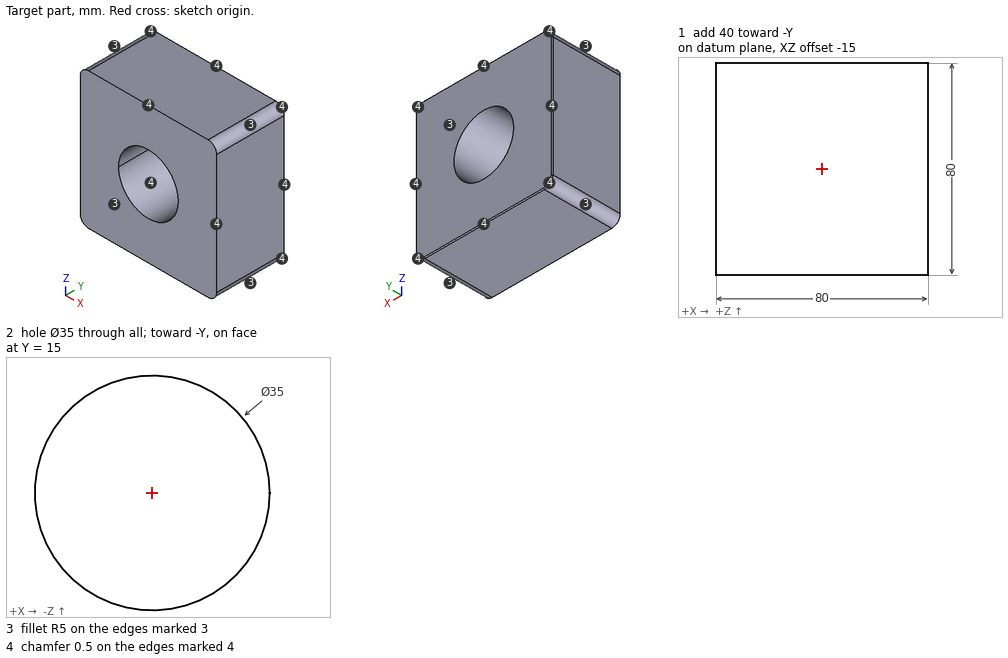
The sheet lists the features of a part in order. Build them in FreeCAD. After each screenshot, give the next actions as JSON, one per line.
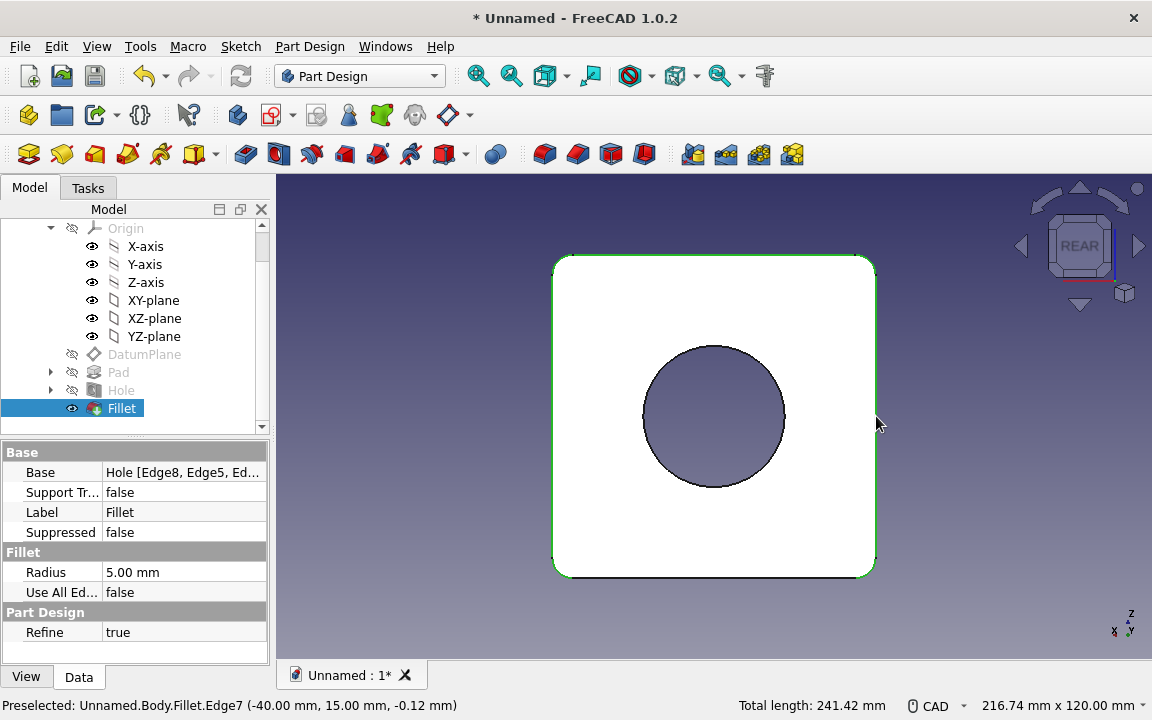
{"action": "left_click", "coordinate": [714, 577], "text": "ctrl"}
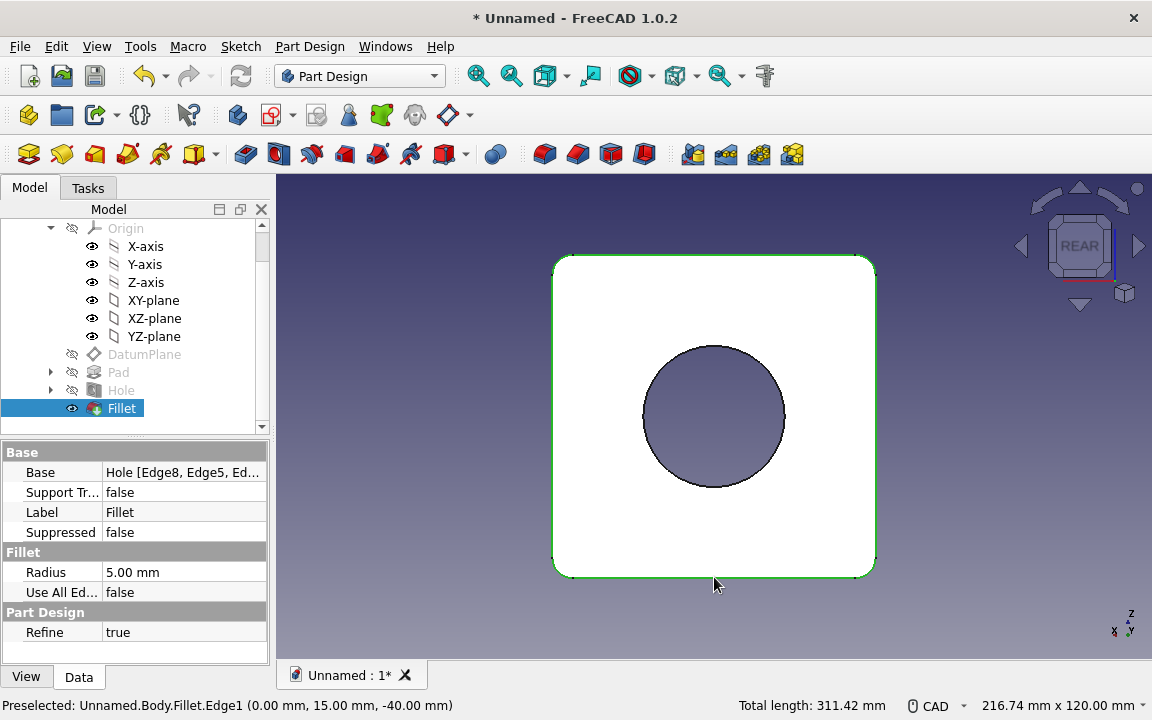
{"action": "left_click", "coordinate": [578, 154]}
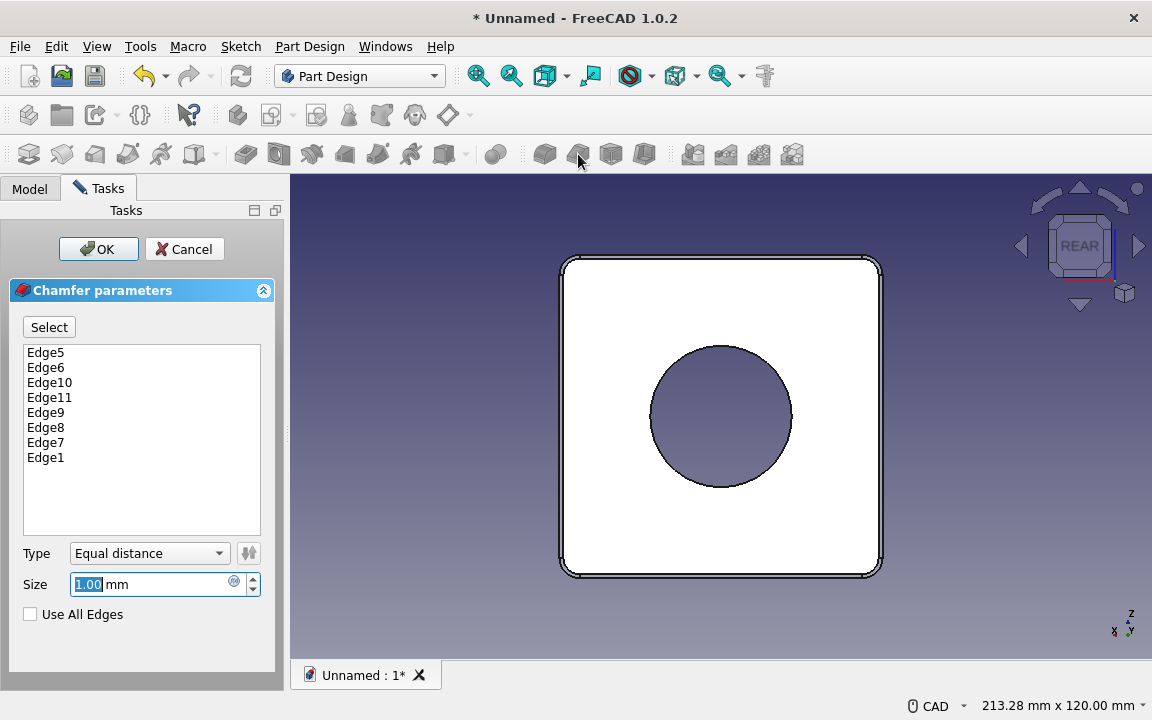
{"action": "type", "text": "0.5"}
{"action": "key", "text": "Tab"}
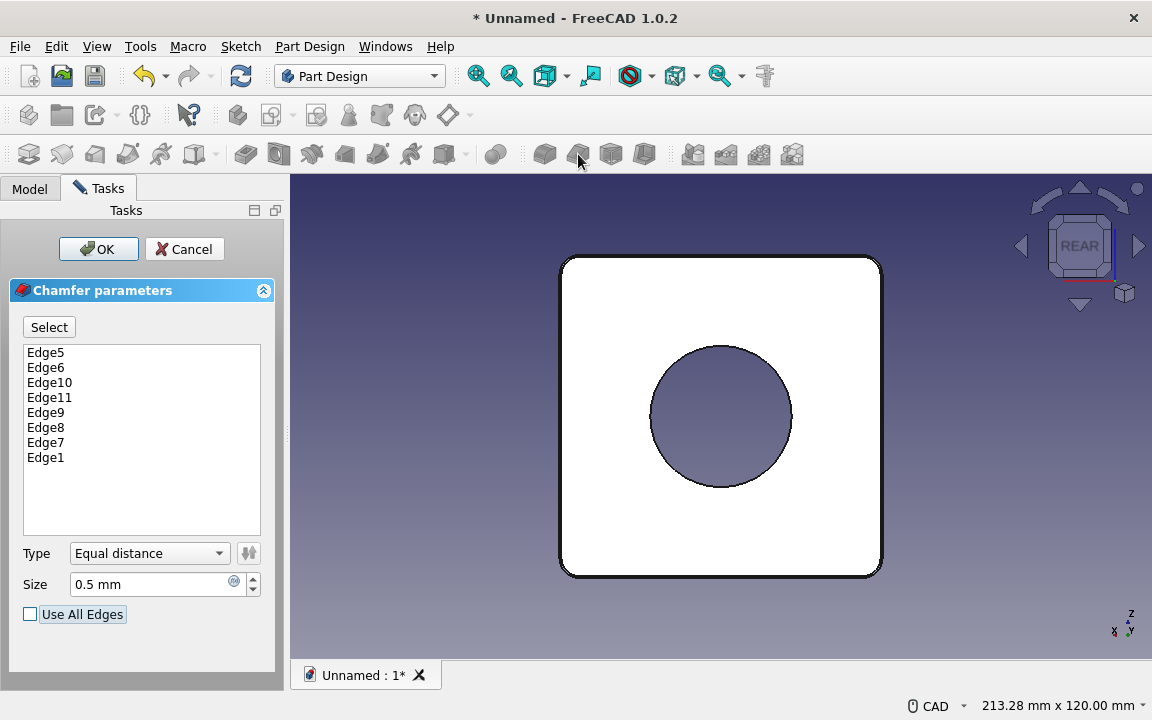
{"action": "left_click", "coordinate": [99, 249]}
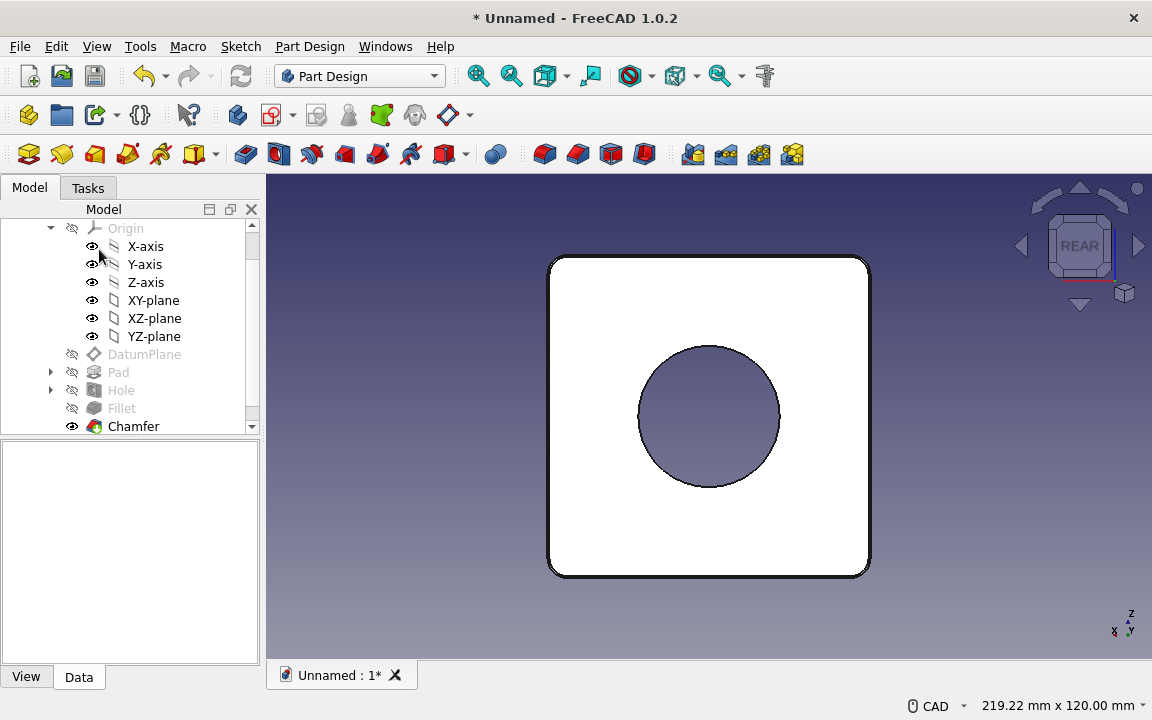
{"action": "key", "text": "0"}